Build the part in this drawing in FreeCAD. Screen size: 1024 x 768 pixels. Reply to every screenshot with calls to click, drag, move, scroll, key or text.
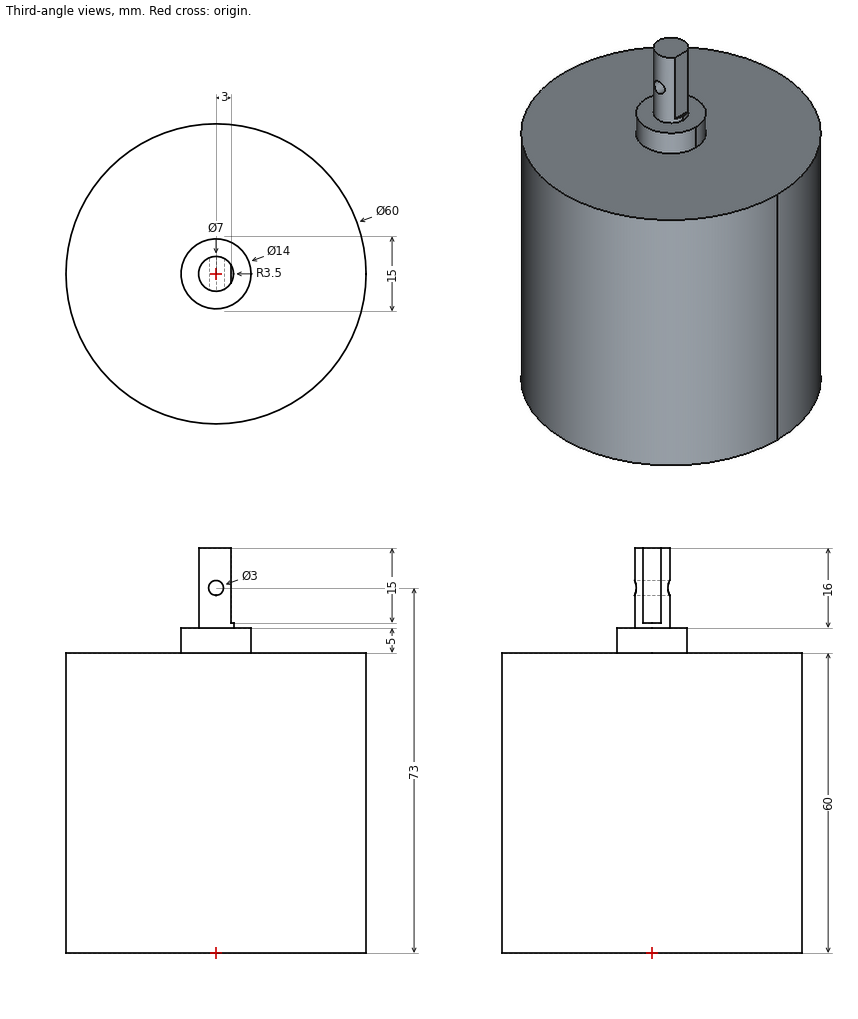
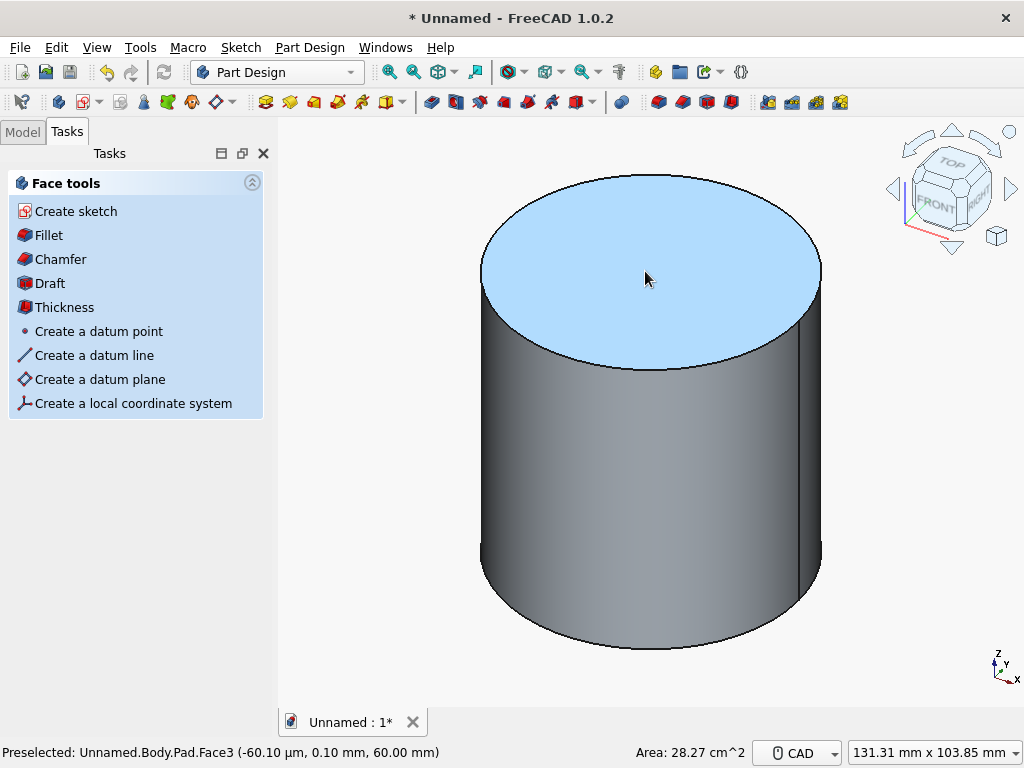
click(84, 102)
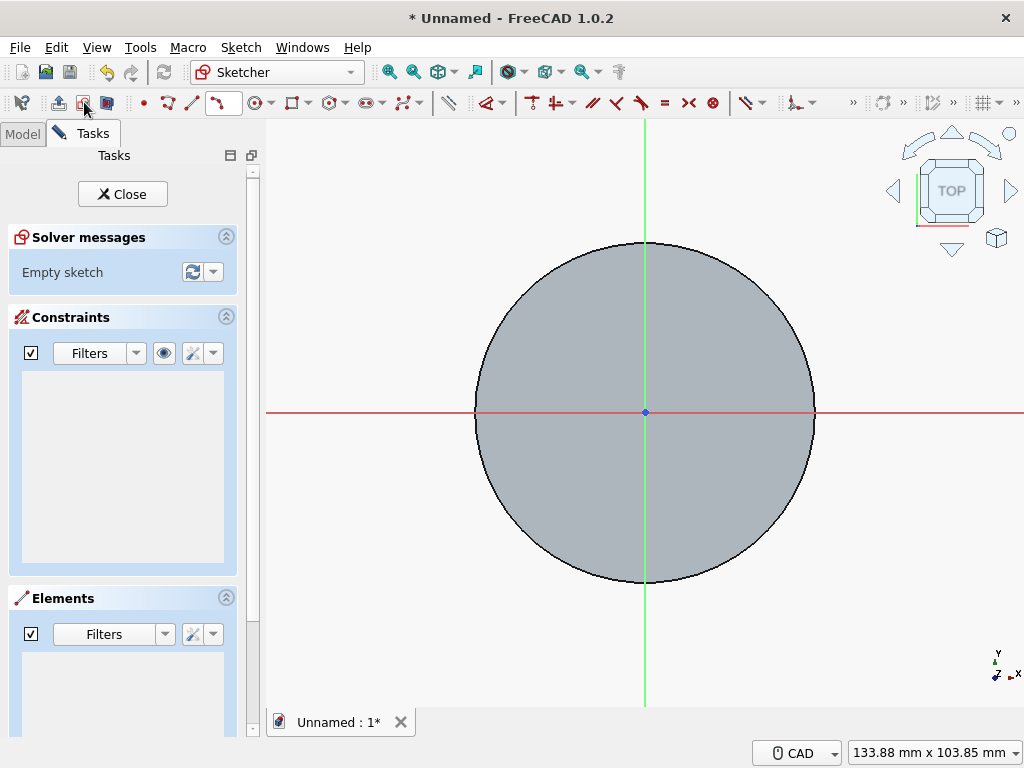
scroll(662, 413, up, 8)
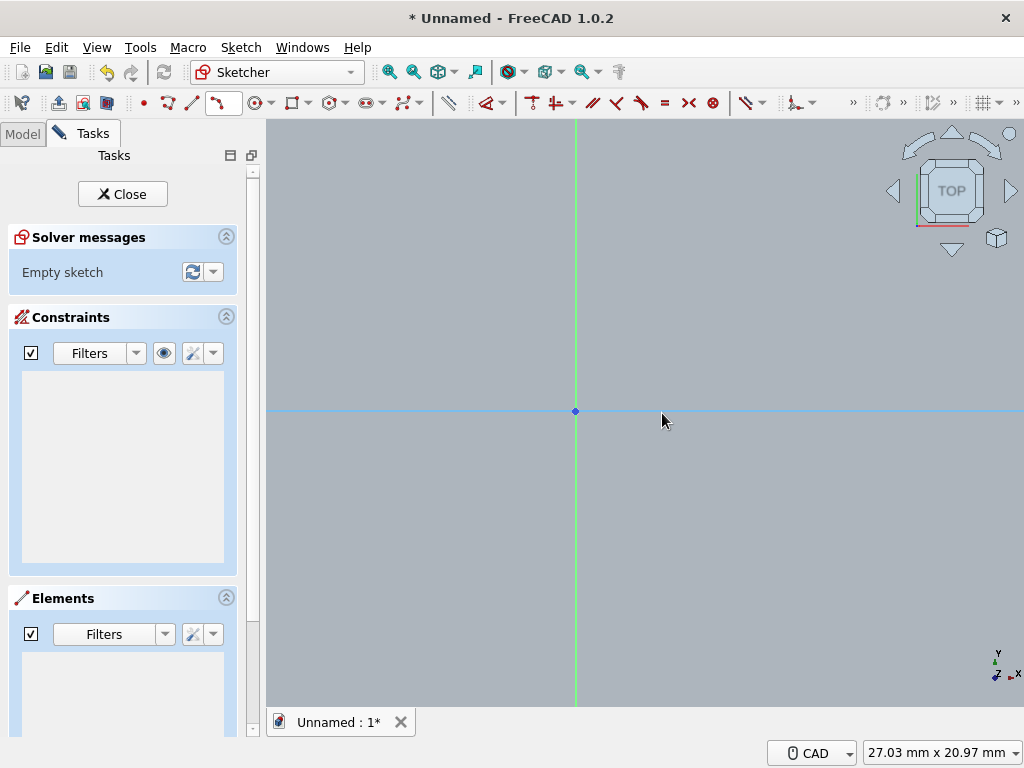
click(256, 104)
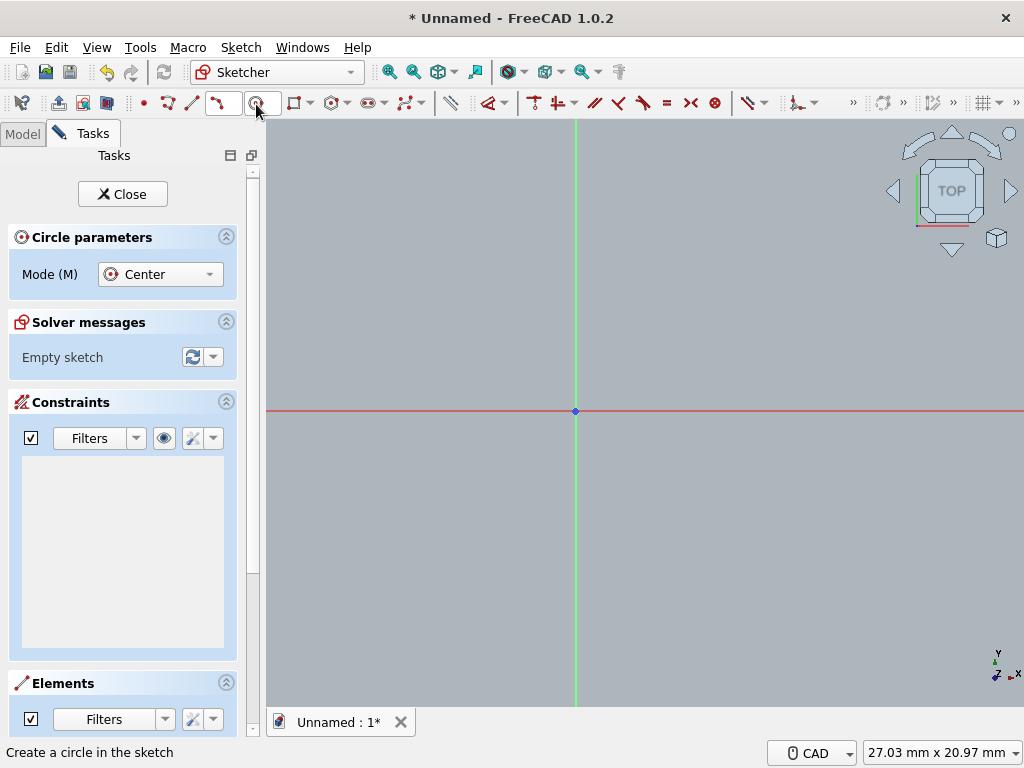
click(576, 411)
move(715, 272)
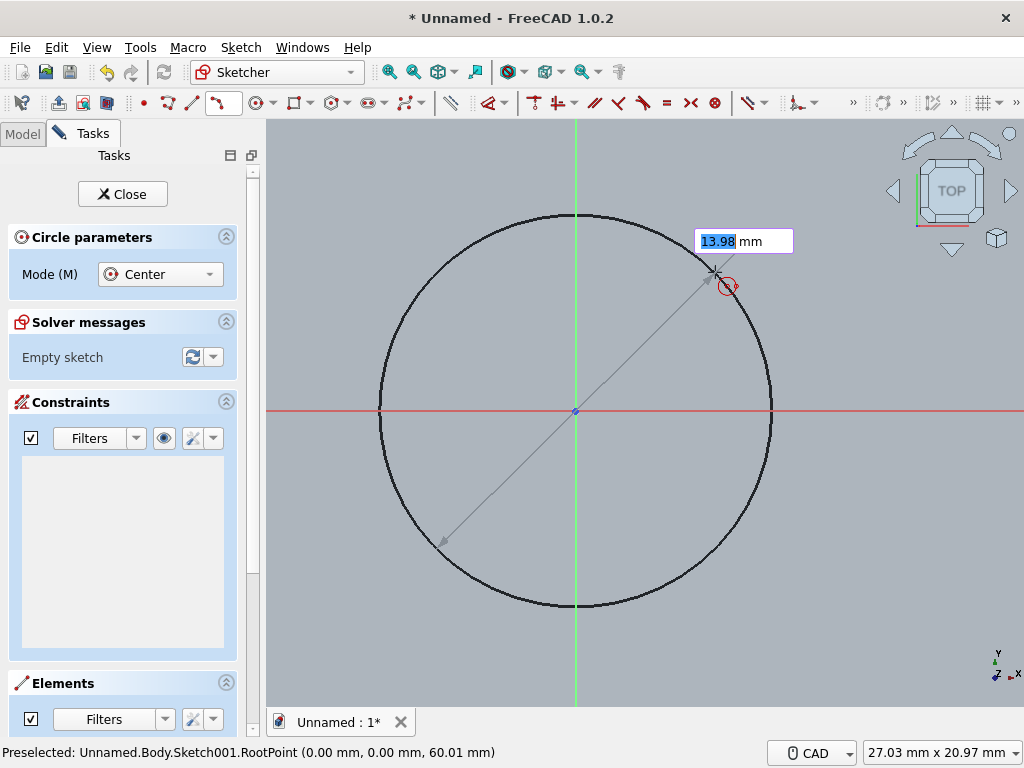
text(14)
key(Return)
key(Escape)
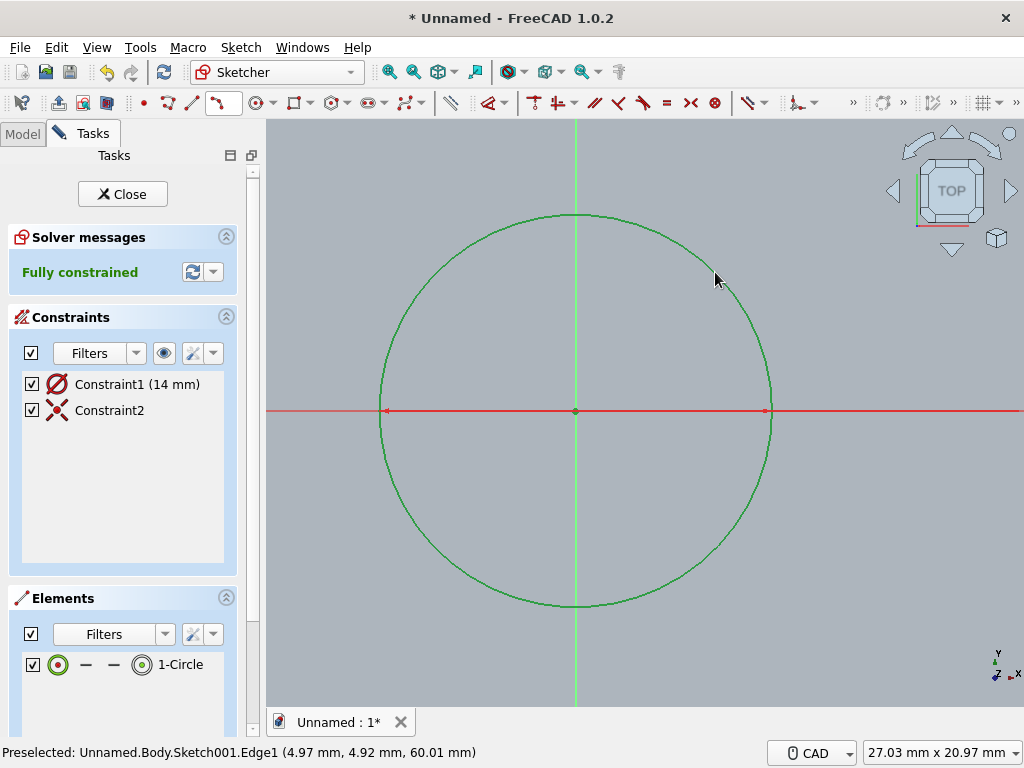
click(123, 194)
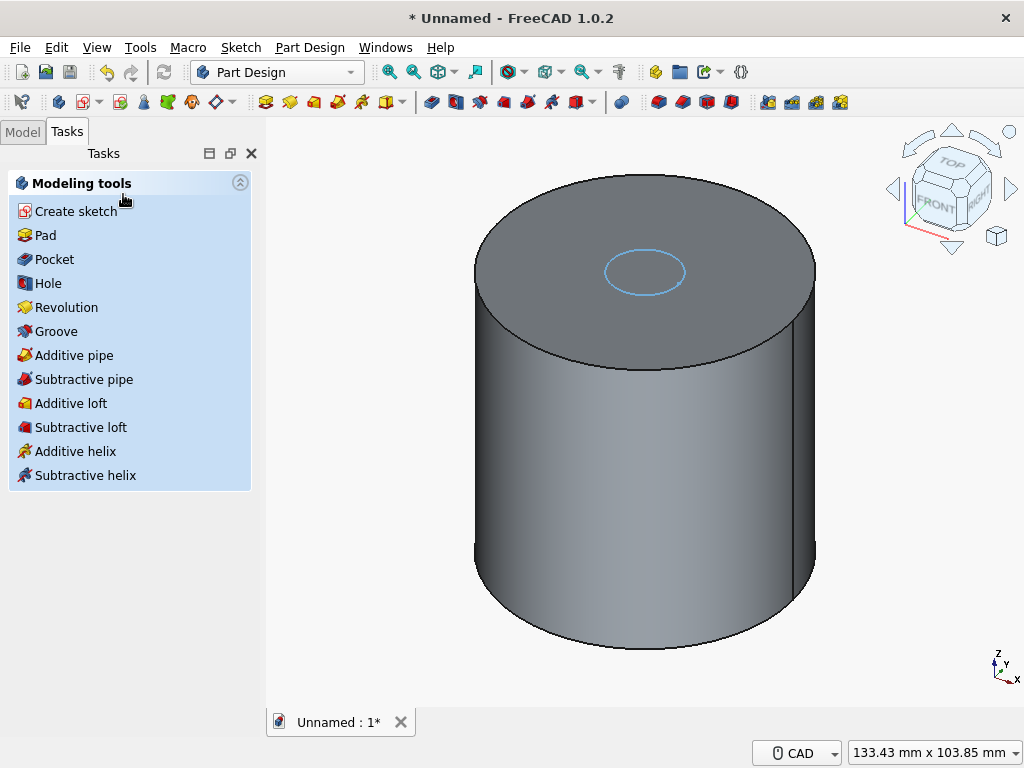
click(266, 102)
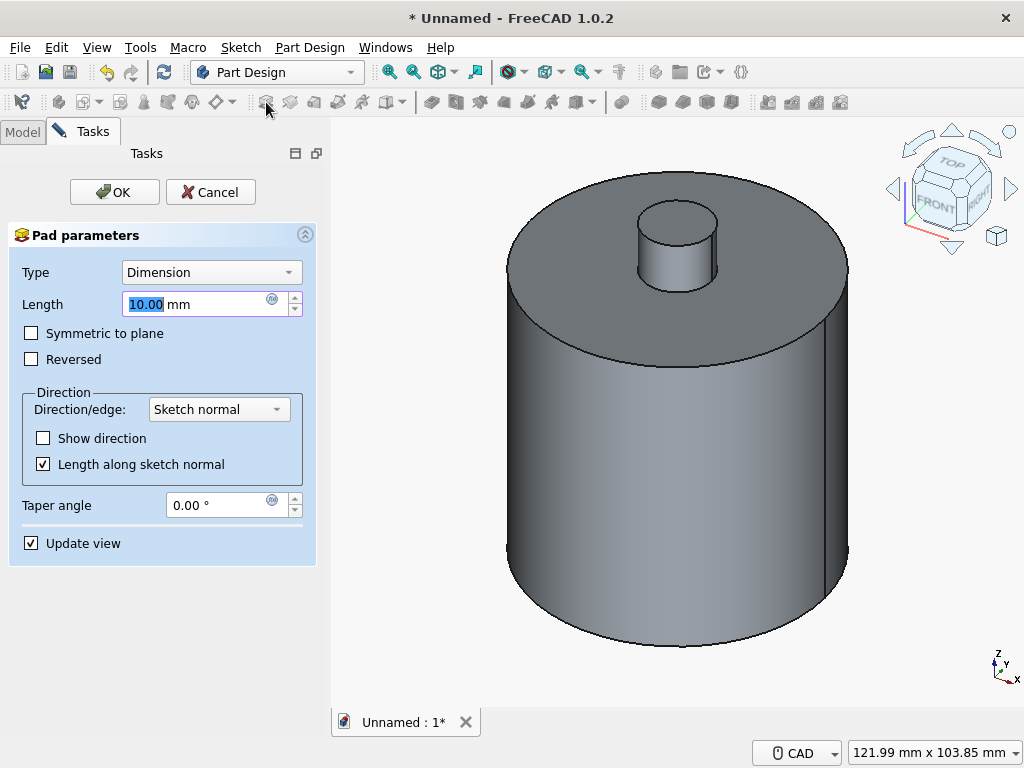
text(5)
key(Tab)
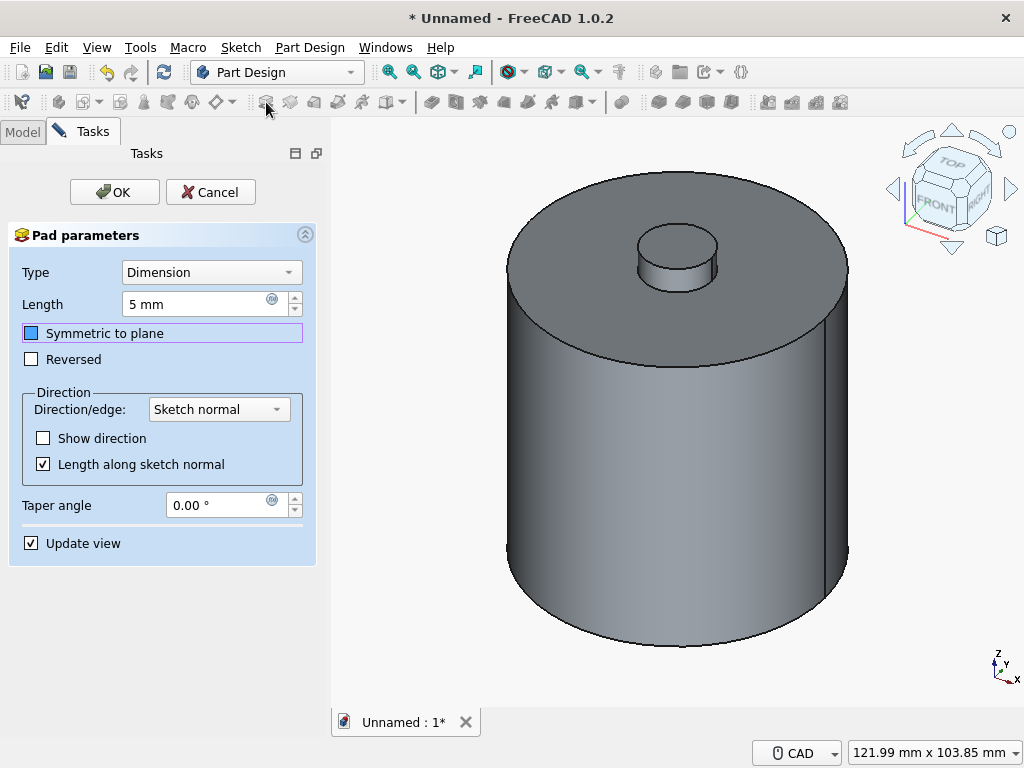
click(115, 192)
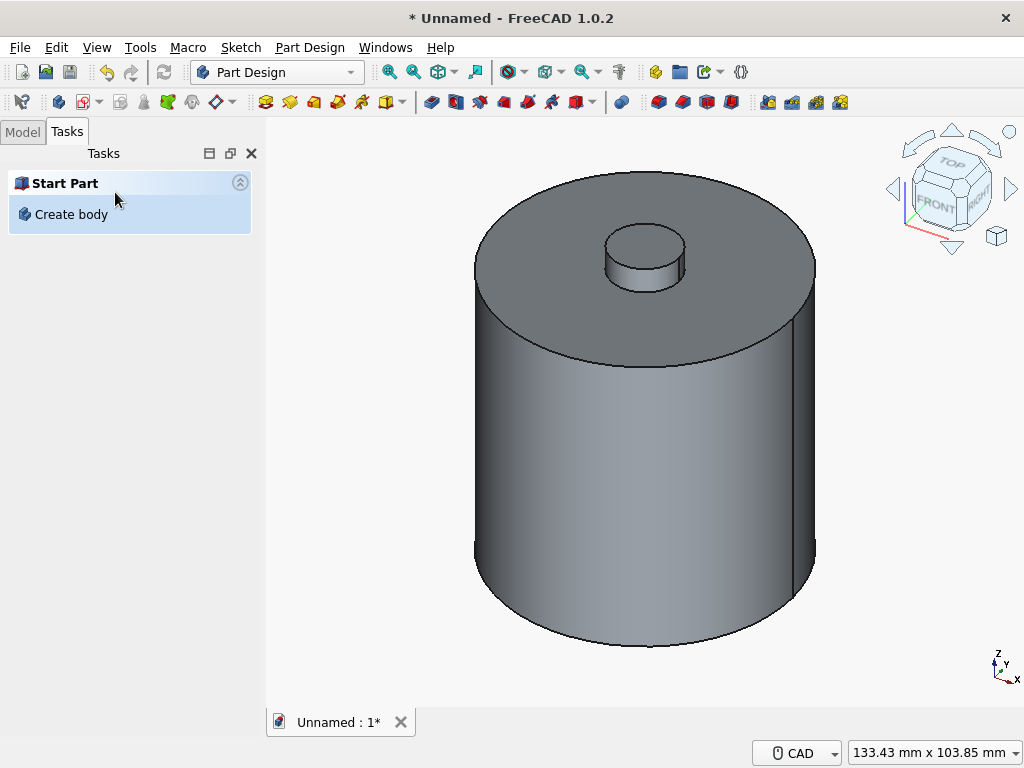
click(390, 72)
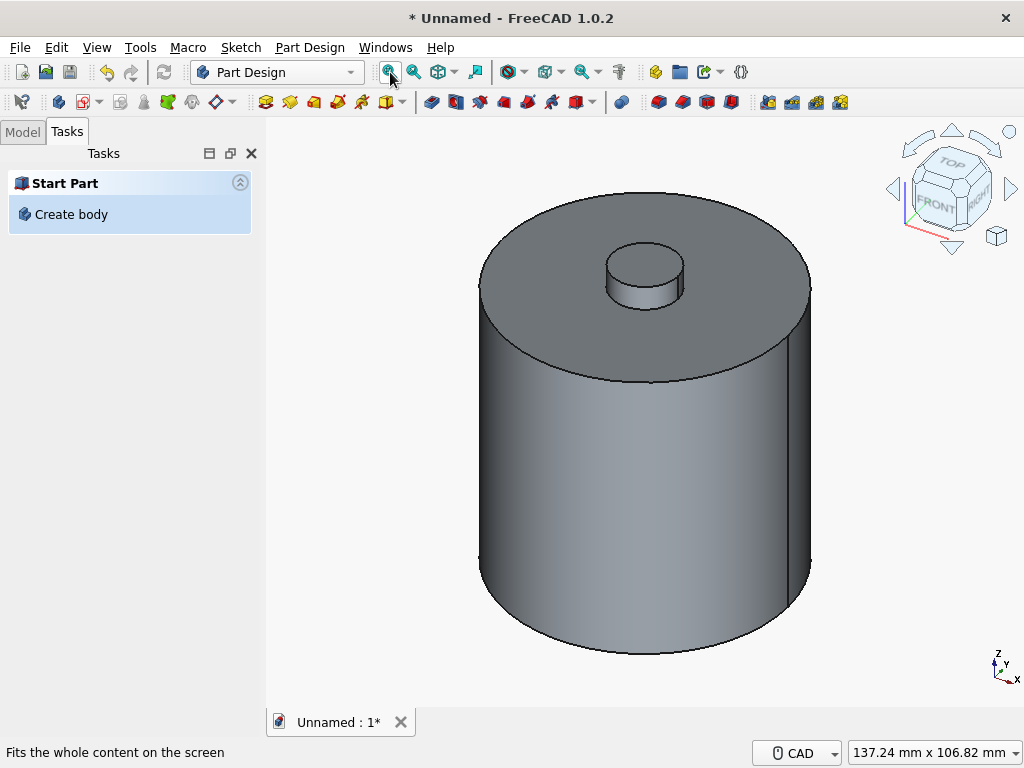
click(645, 264)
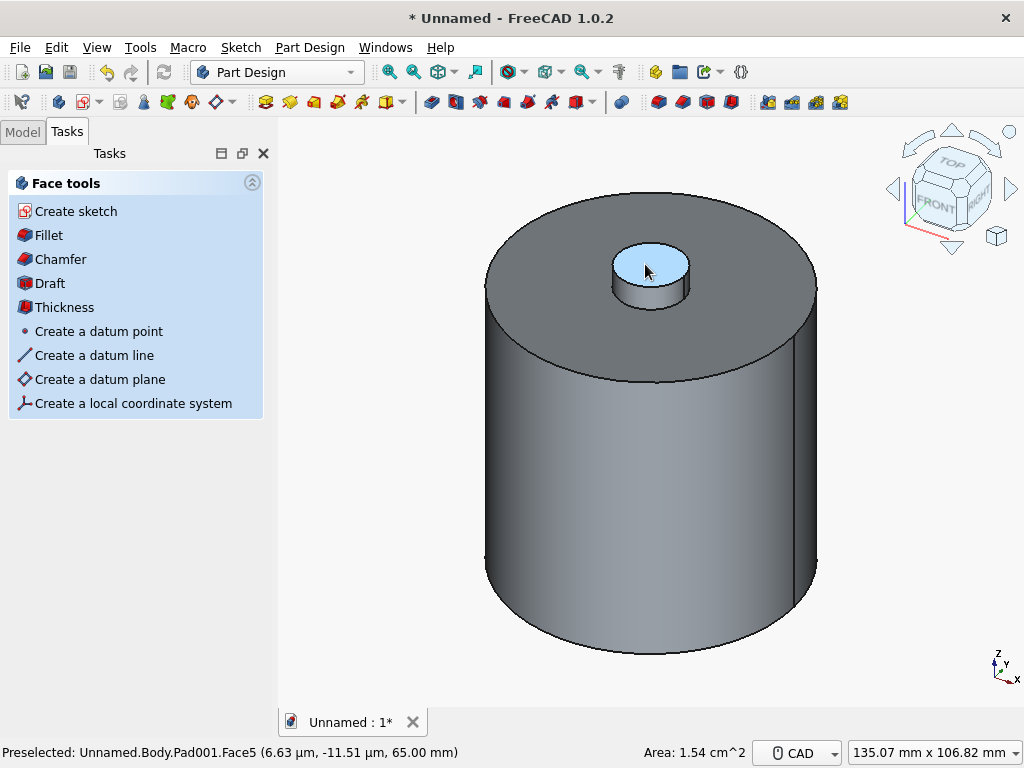
click(84, 102)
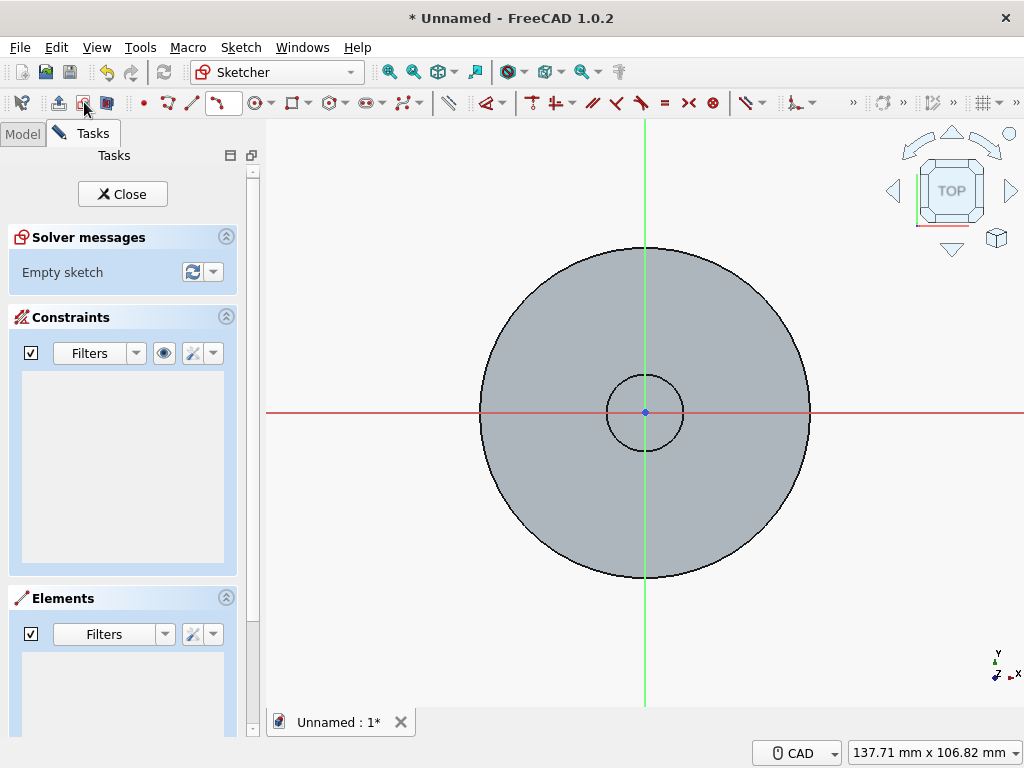
scroll(654, 413, up, 11)